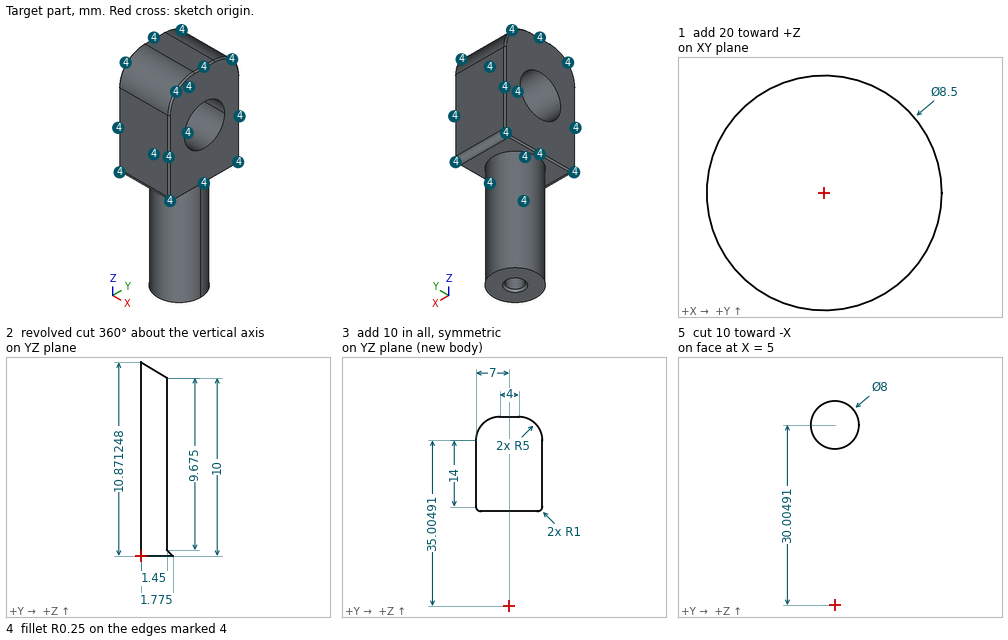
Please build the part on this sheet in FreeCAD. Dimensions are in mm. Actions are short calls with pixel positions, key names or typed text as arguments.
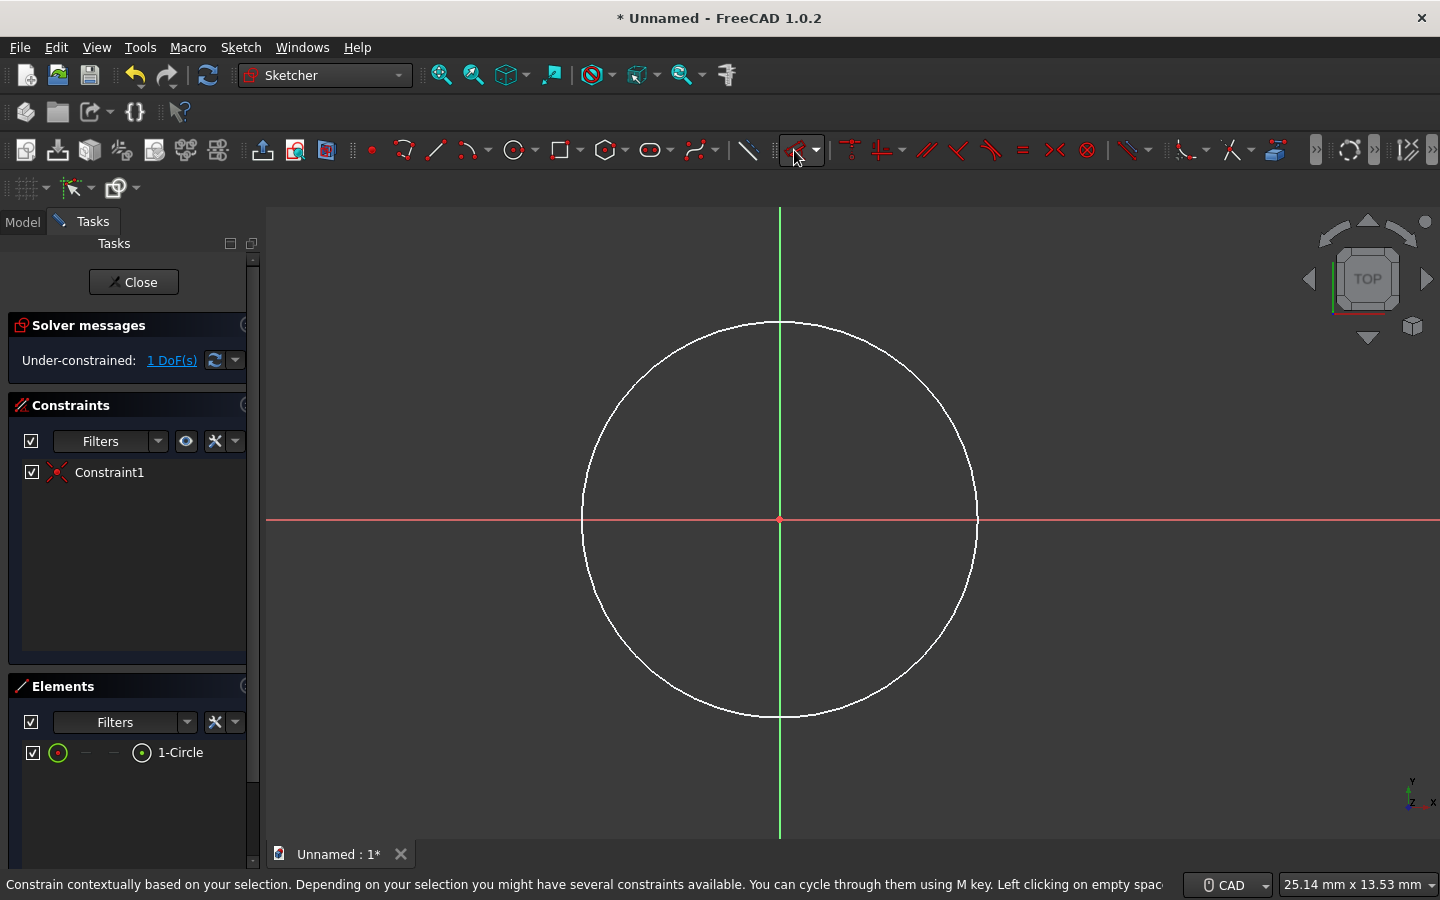
click(919, 379)
click(942, 356)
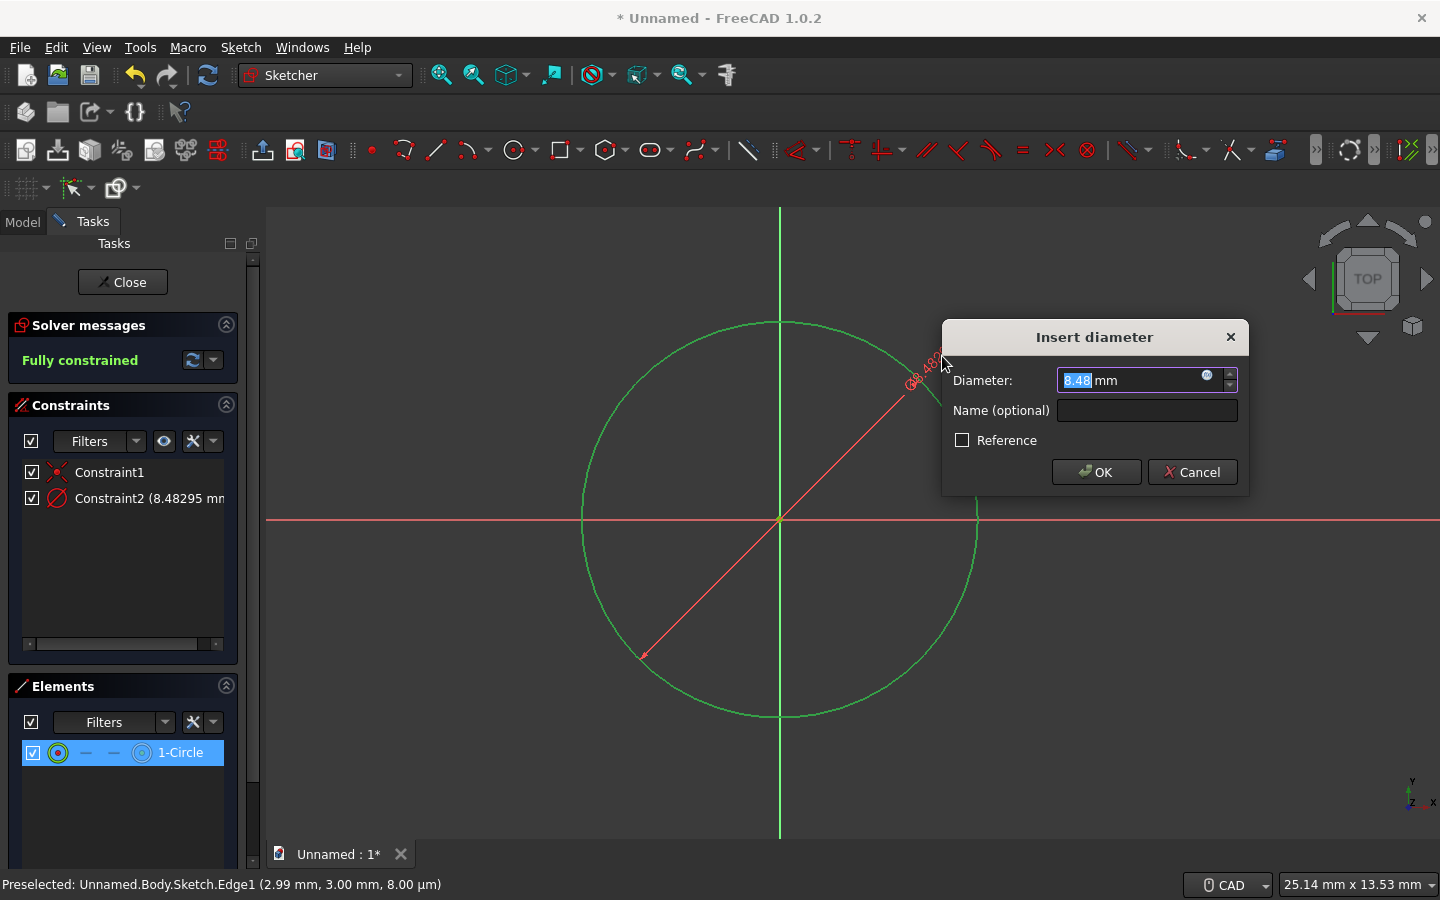
text(8.5)
key(Return)
key(Escape)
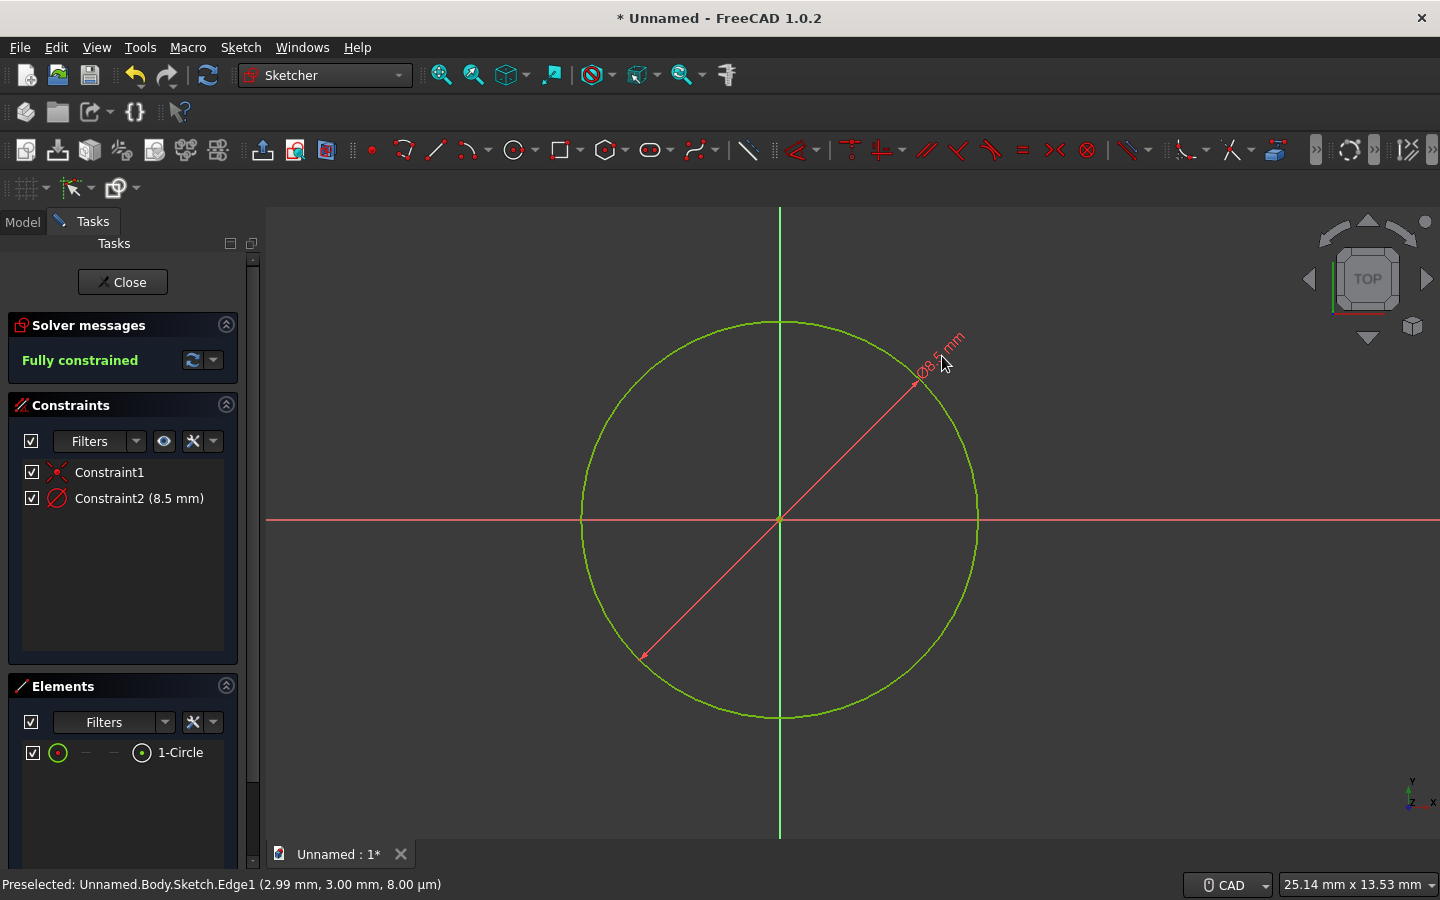
click(123, 282)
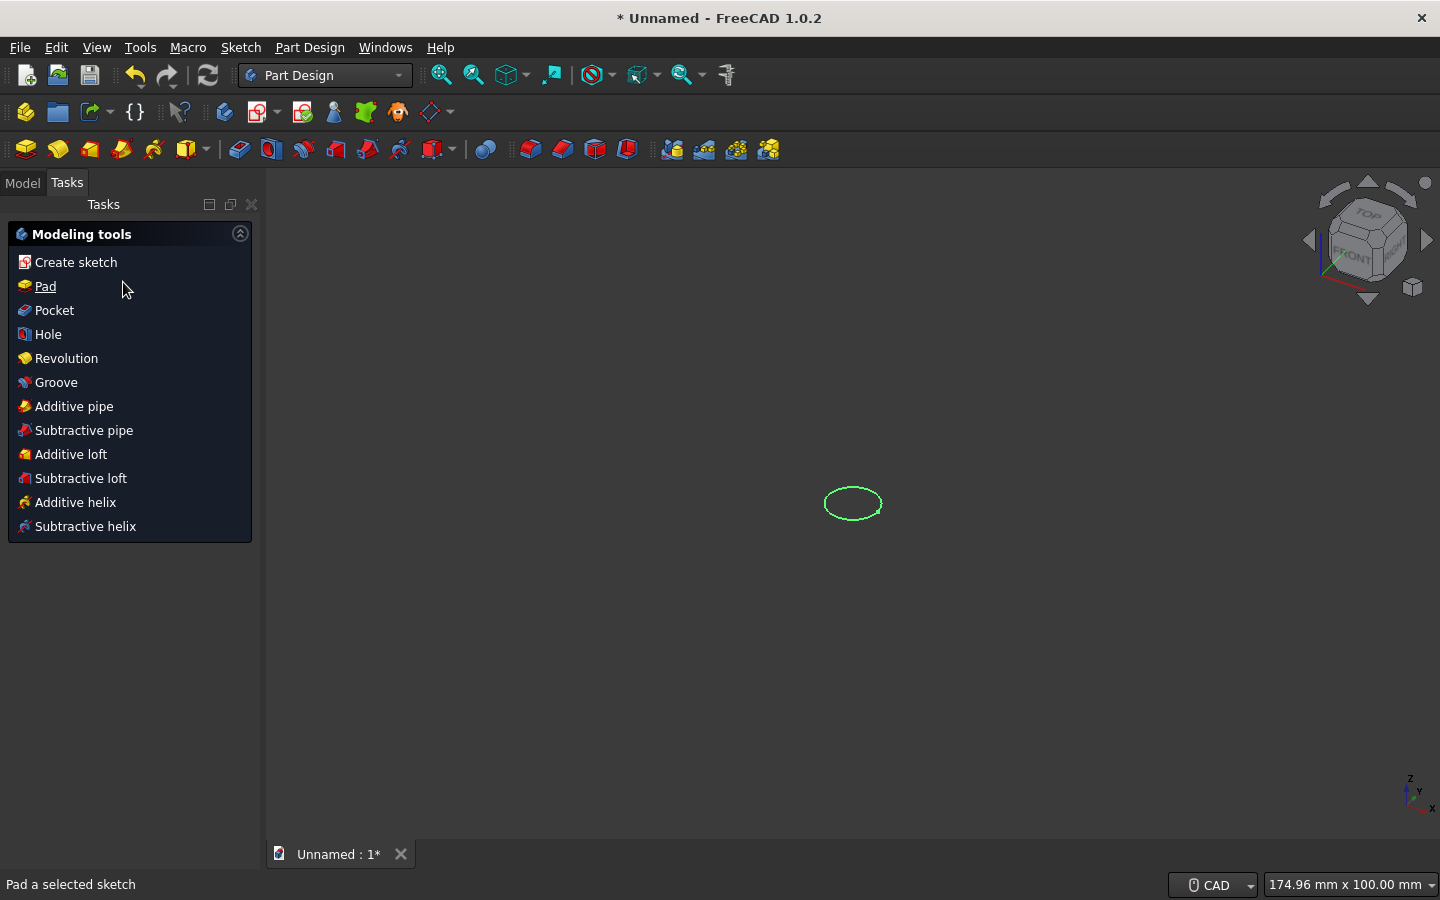
click(26, 150)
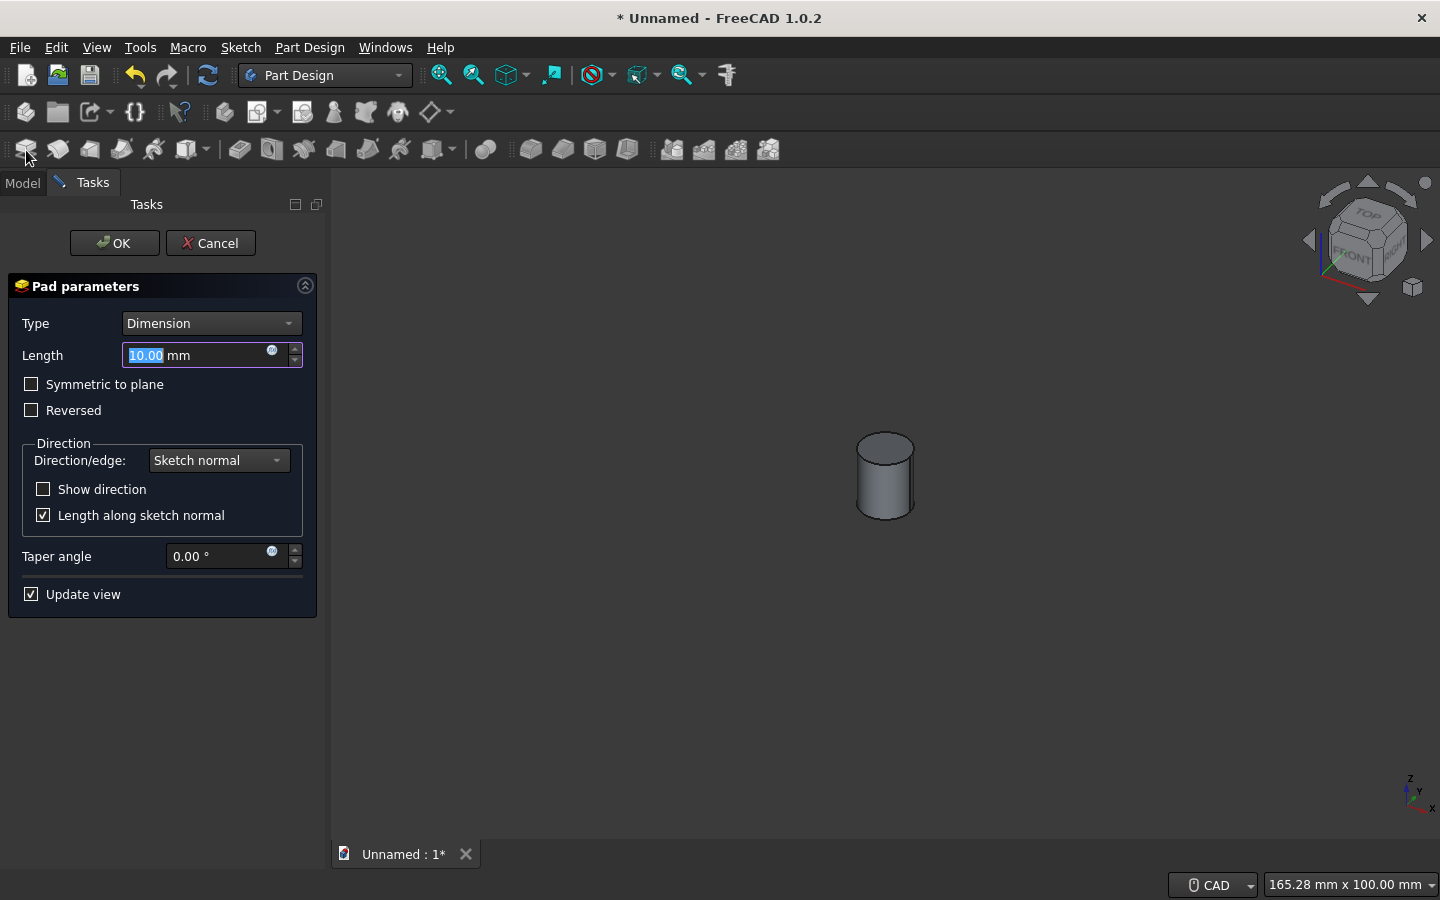
text(20)
key(Tab)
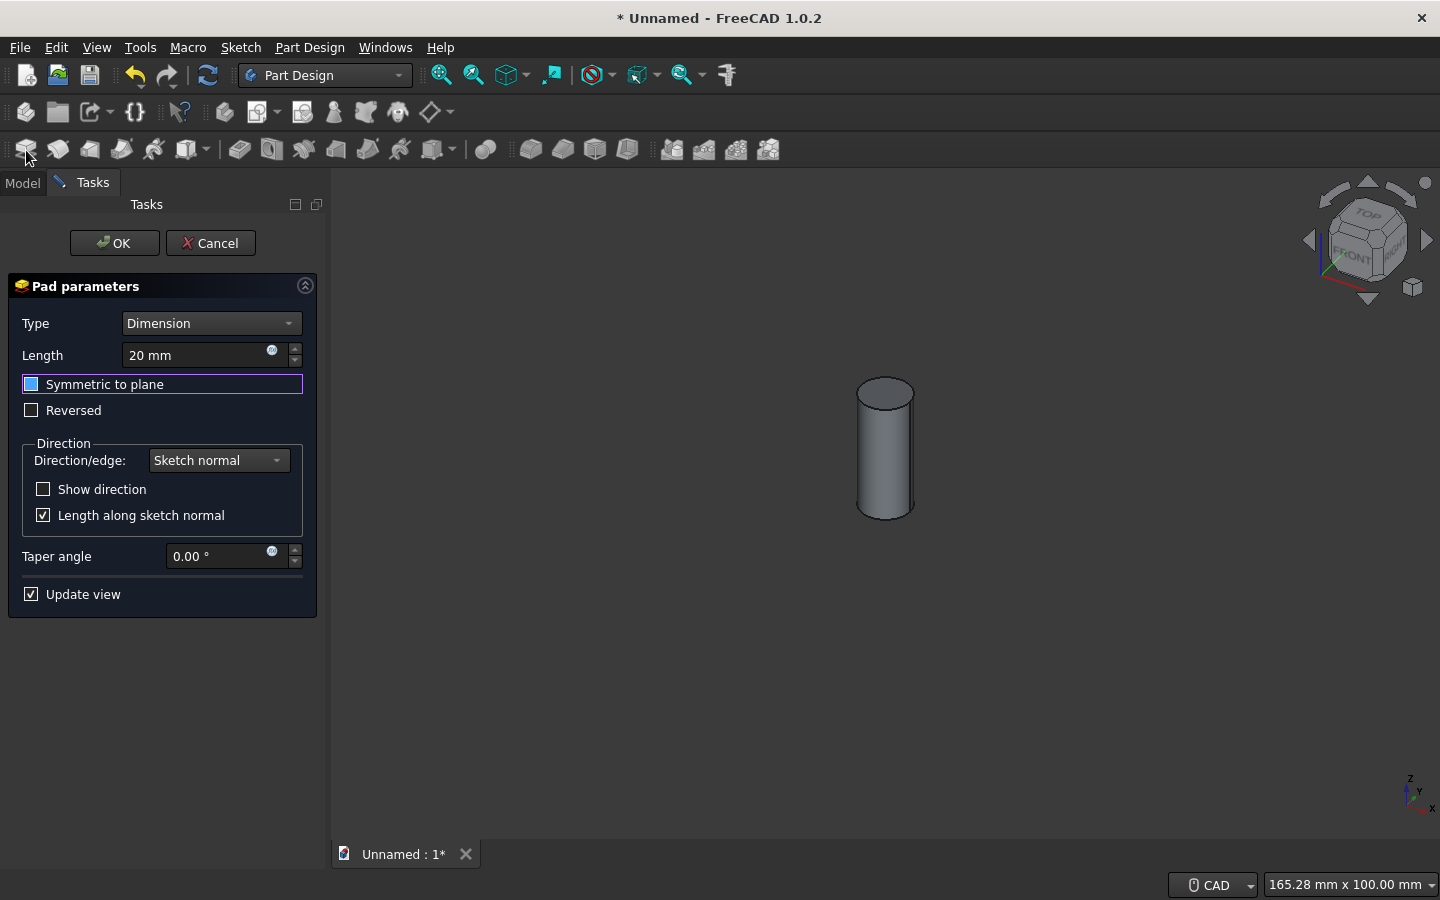
click(115, 243)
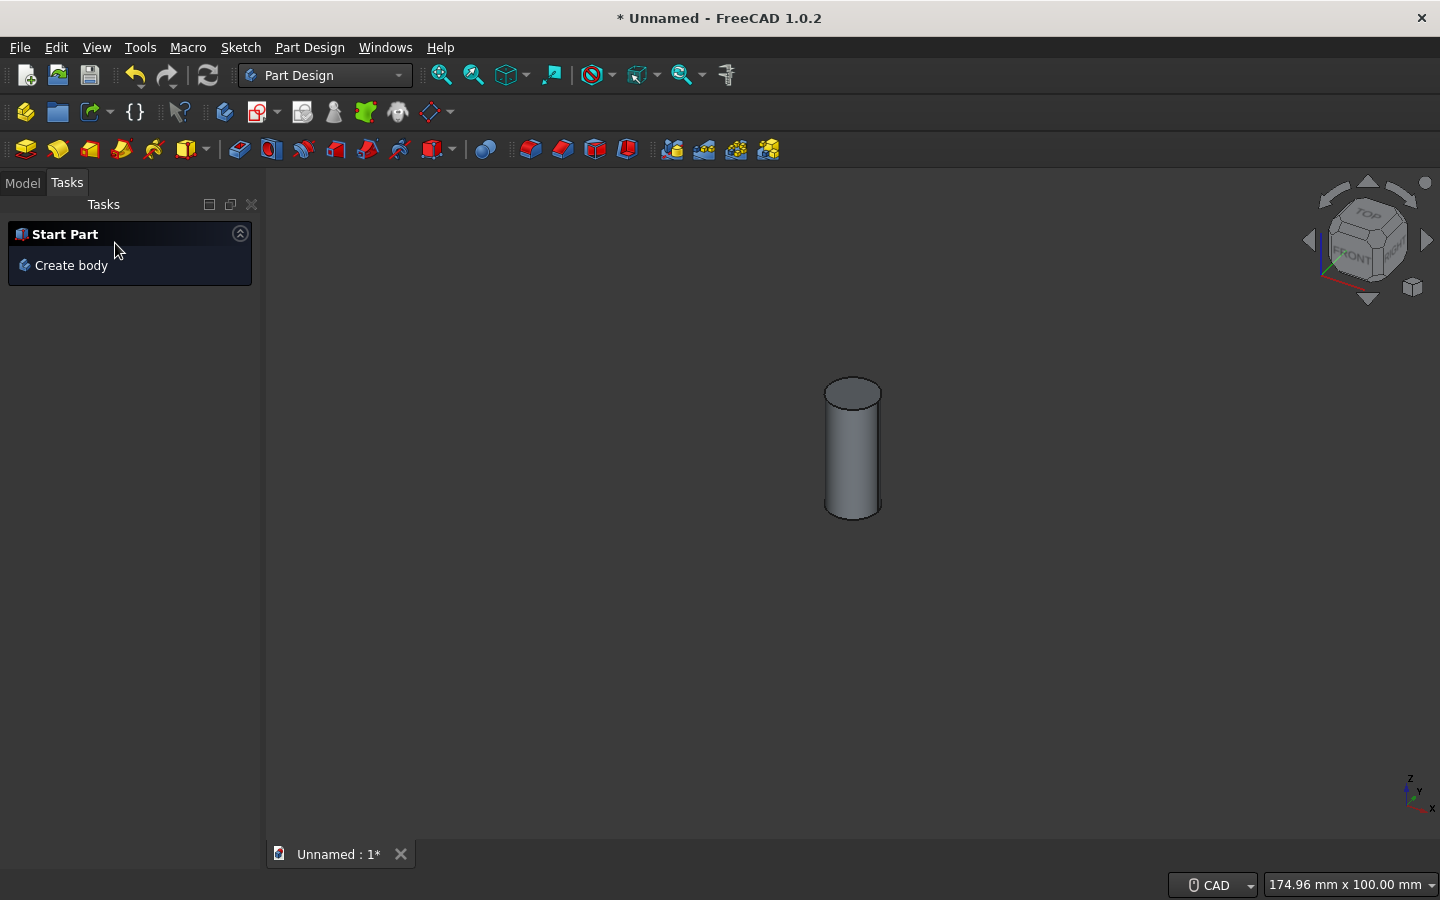
key(v)
key(f)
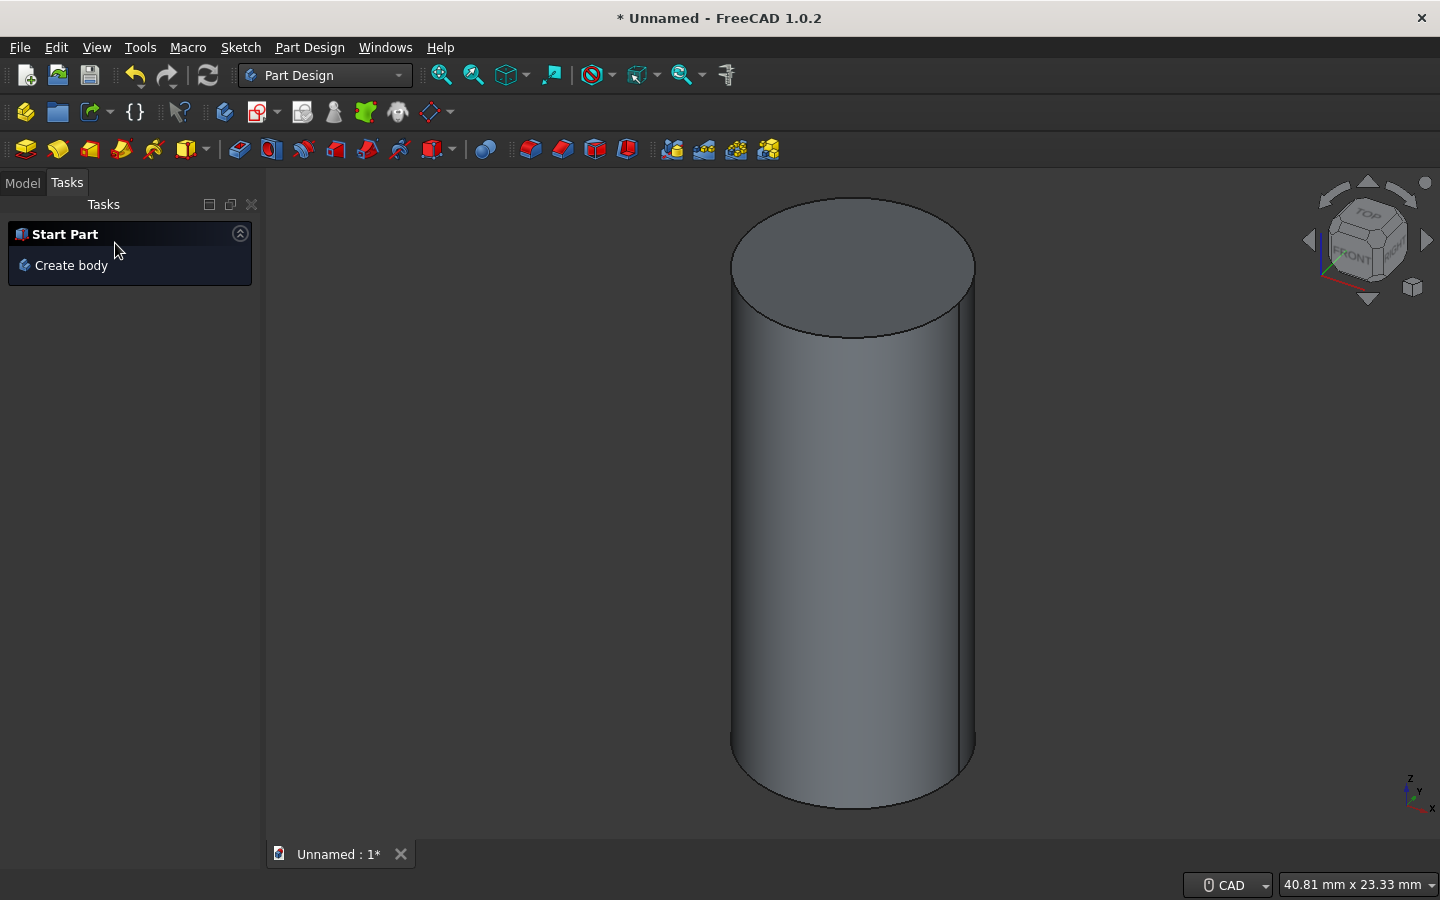
click(258, 112)